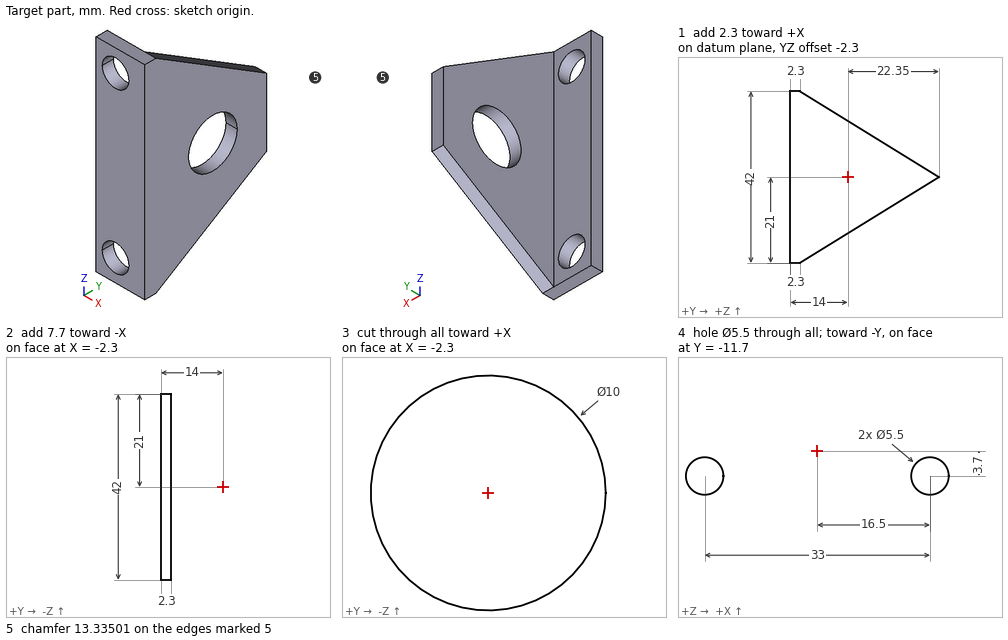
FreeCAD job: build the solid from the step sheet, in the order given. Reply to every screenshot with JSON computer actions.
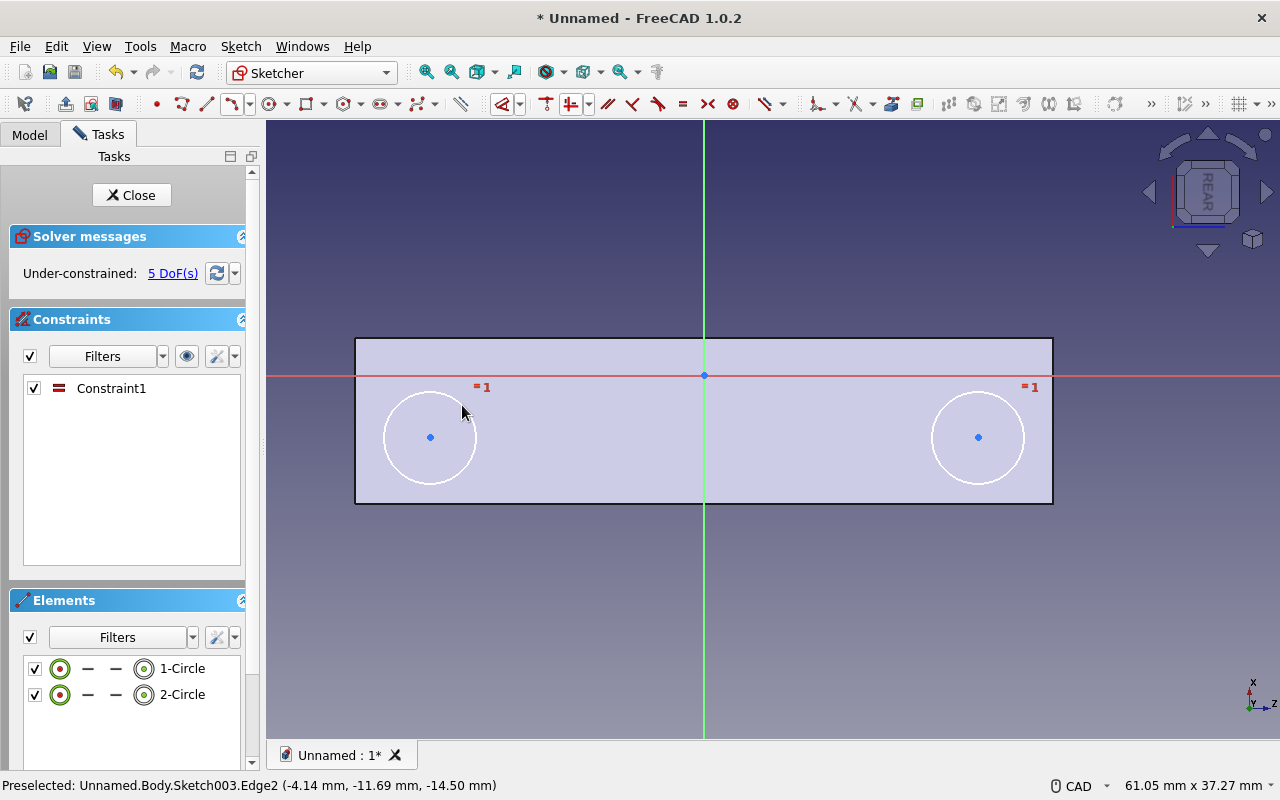
{"action": "left_click", "coordinate": [978, 438]}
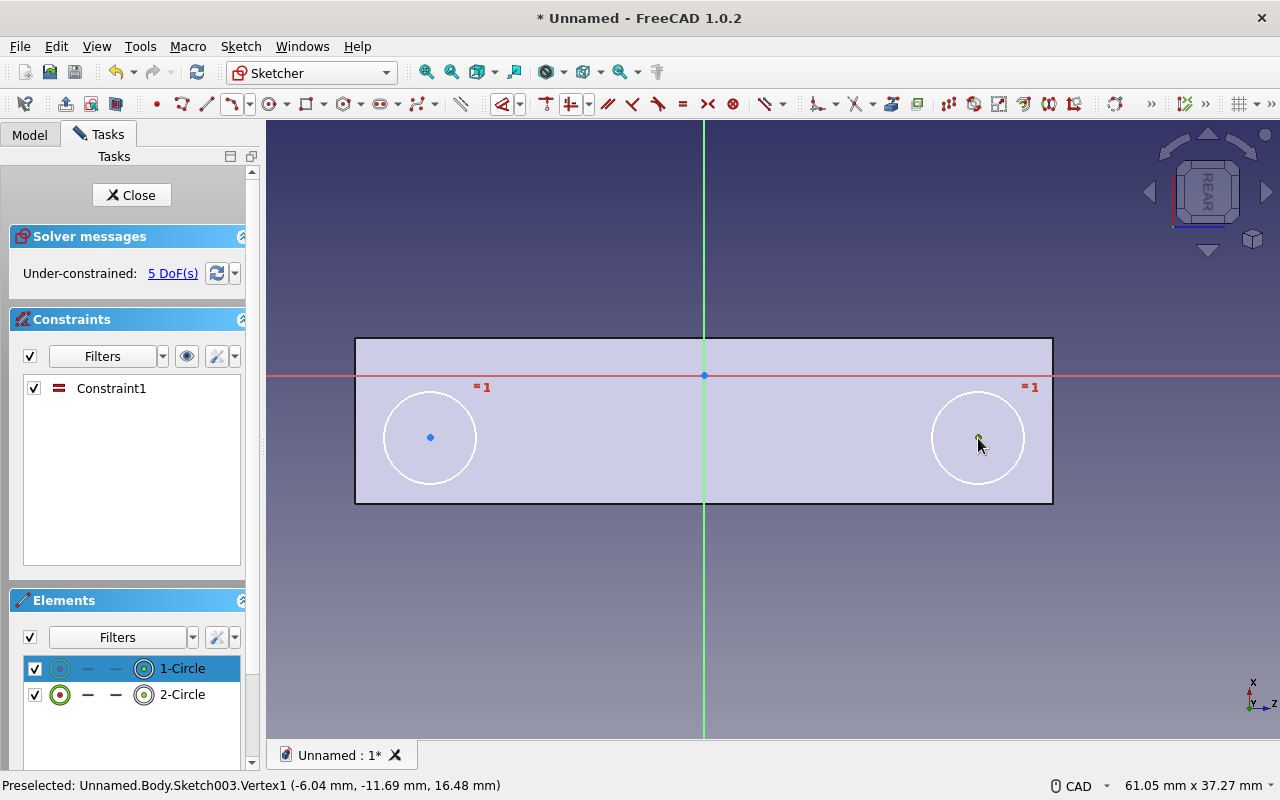
{"action": "left_click", "coordinate": [430, 438]}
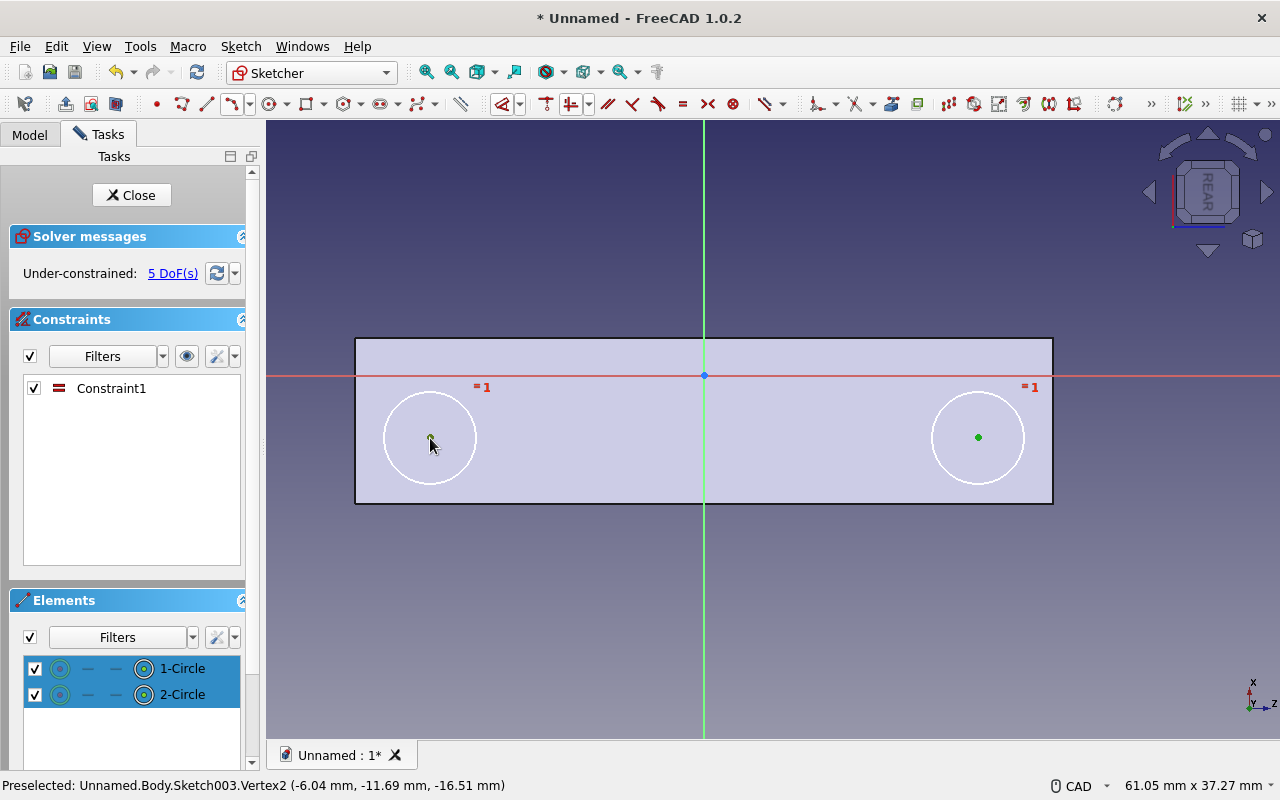
{"action": "key", "text": "h"}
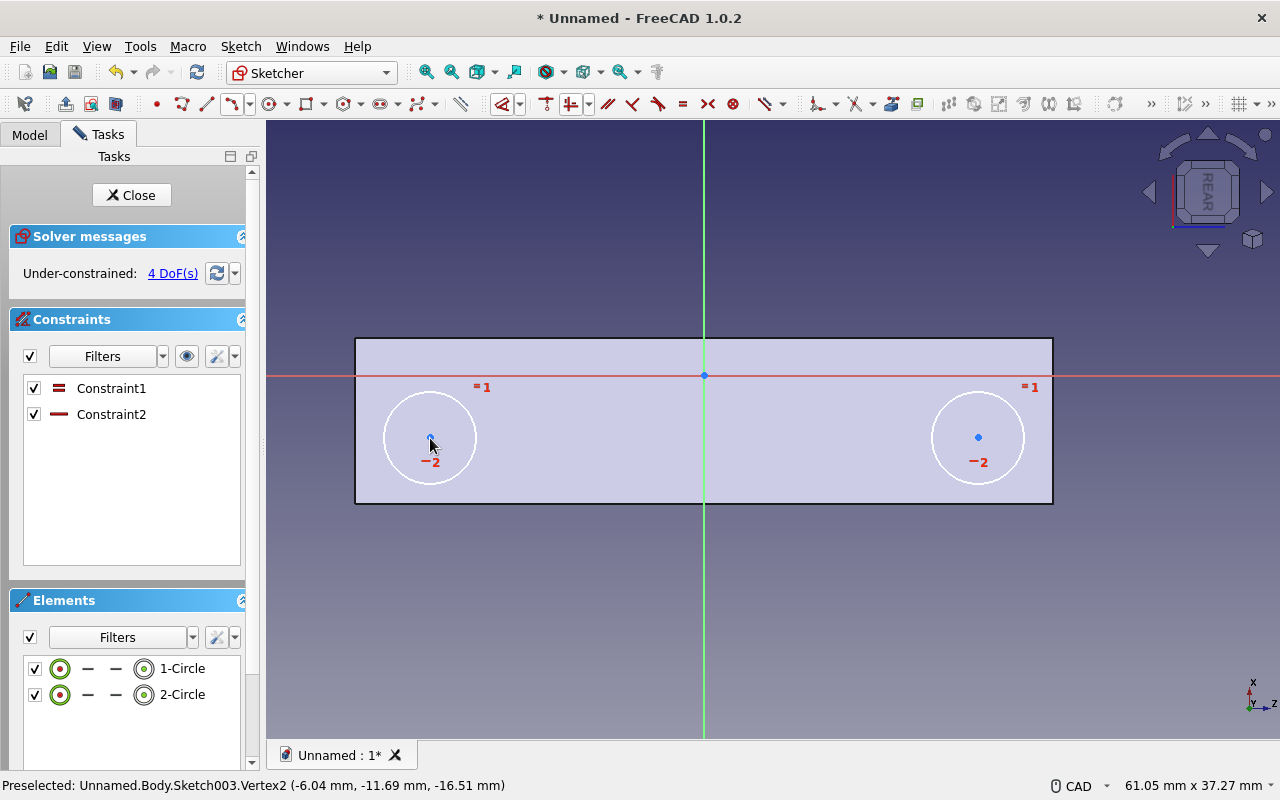
{"action": "left_click", "coordinate": [1010, 405]}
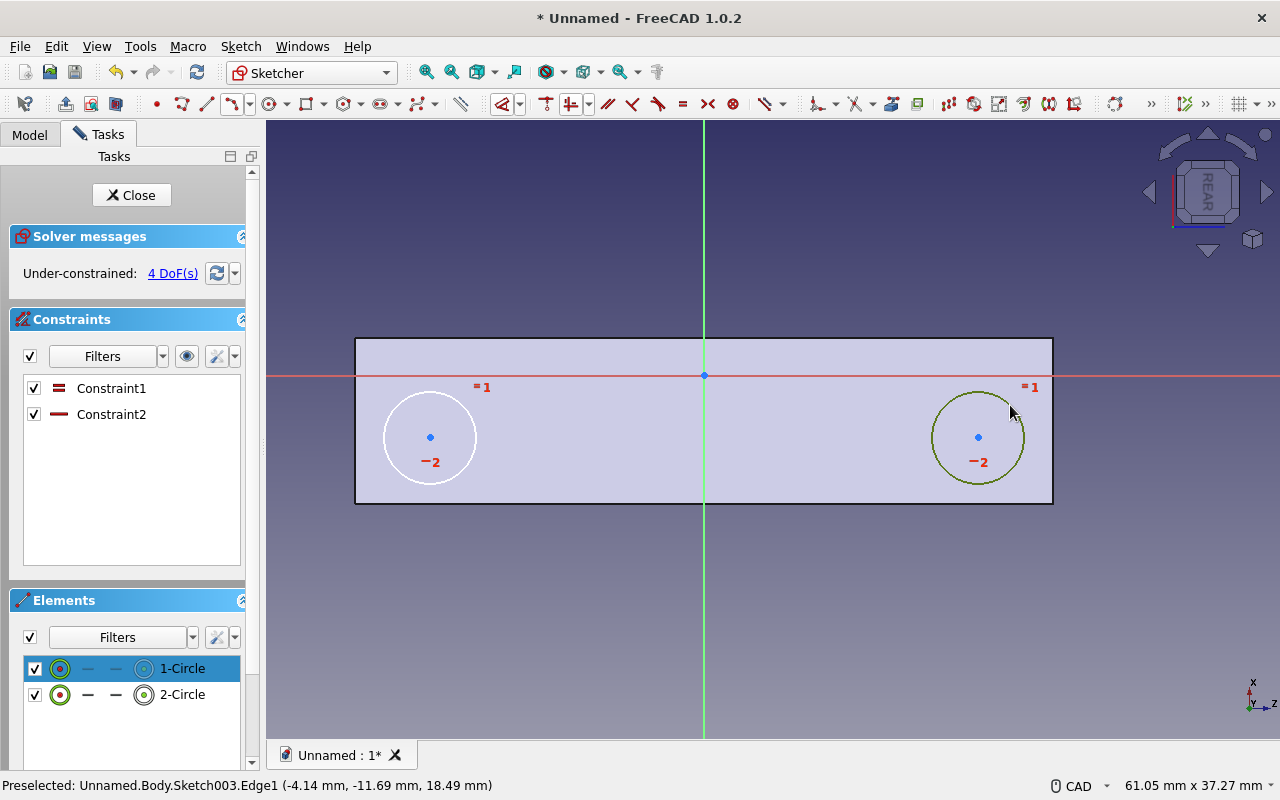
{"action": "left_click", "coordinate": [520, 104]}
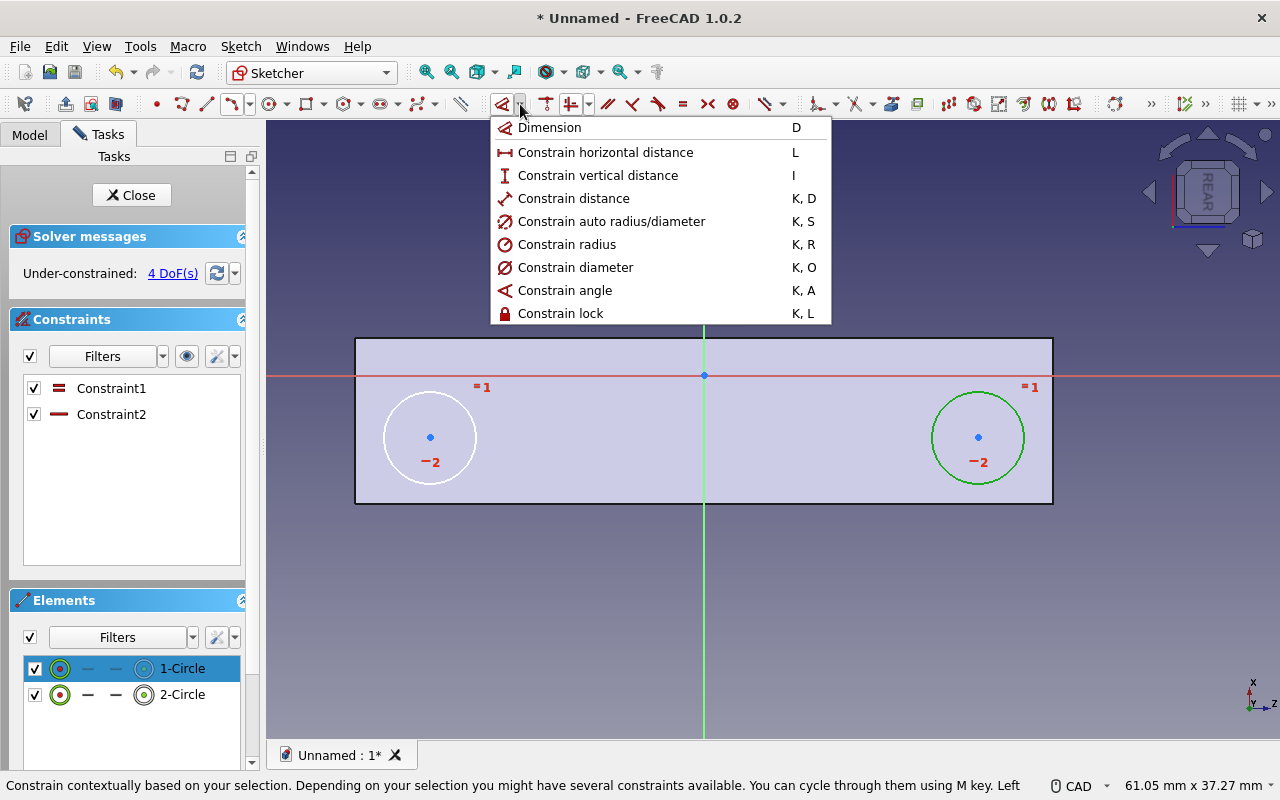
{"action": "left_click", "coordinate": [661, 268]}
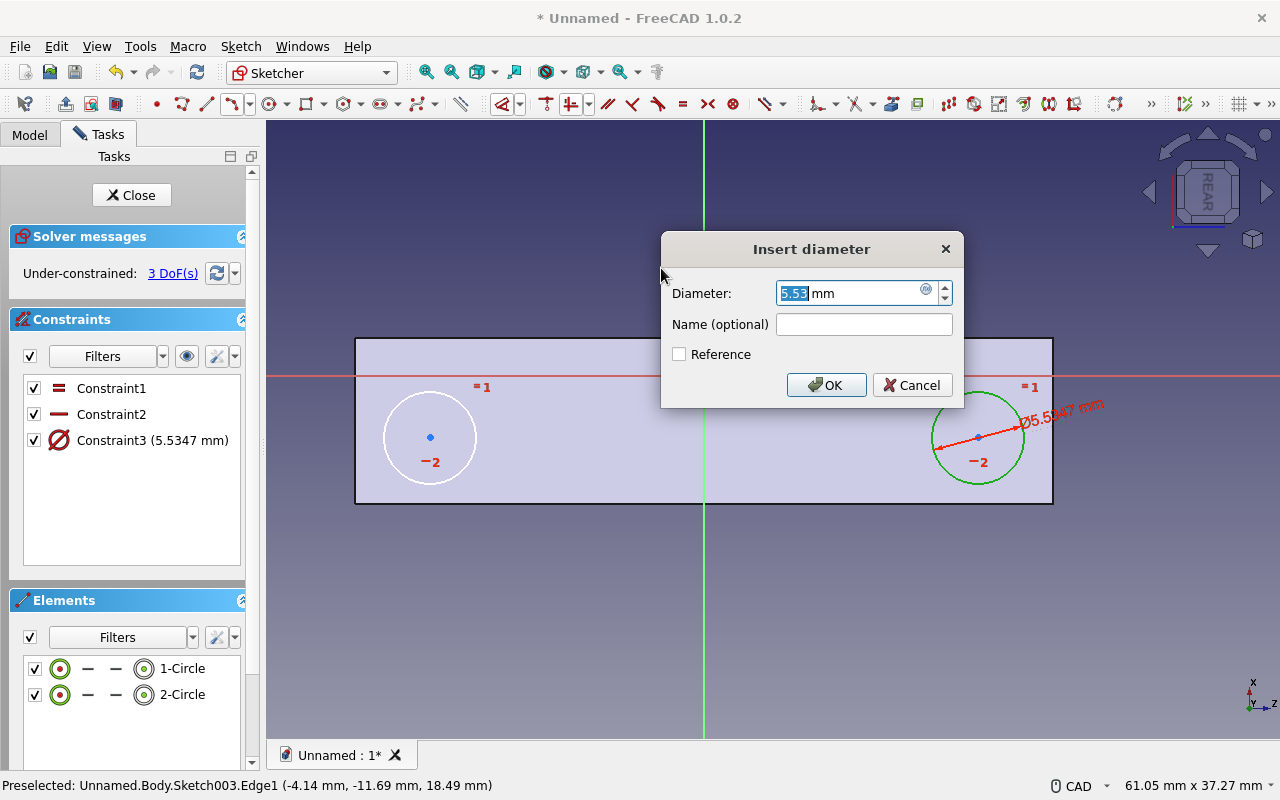
{"action": "type", "text": "5.5"}
{"action": "key", "text": "Return"}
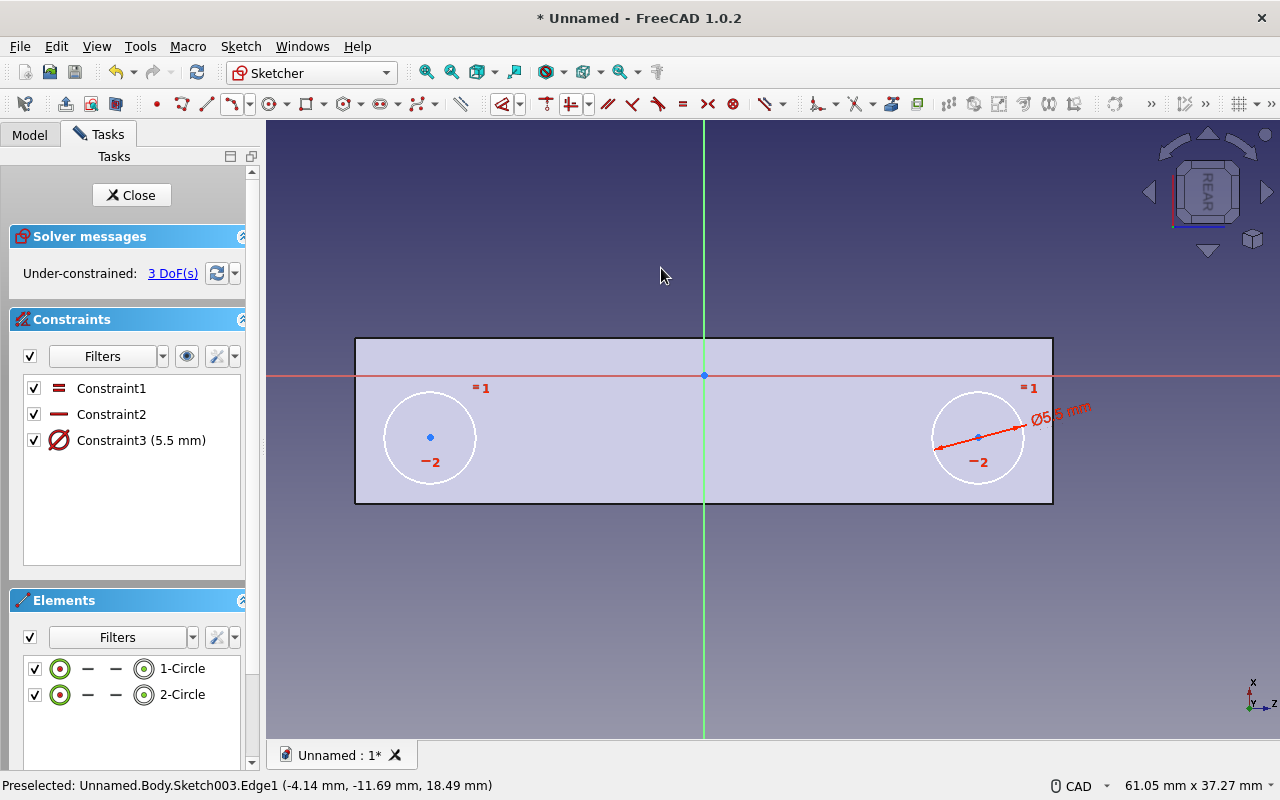
{"action": "left_click", "coordinate": [978, 438]}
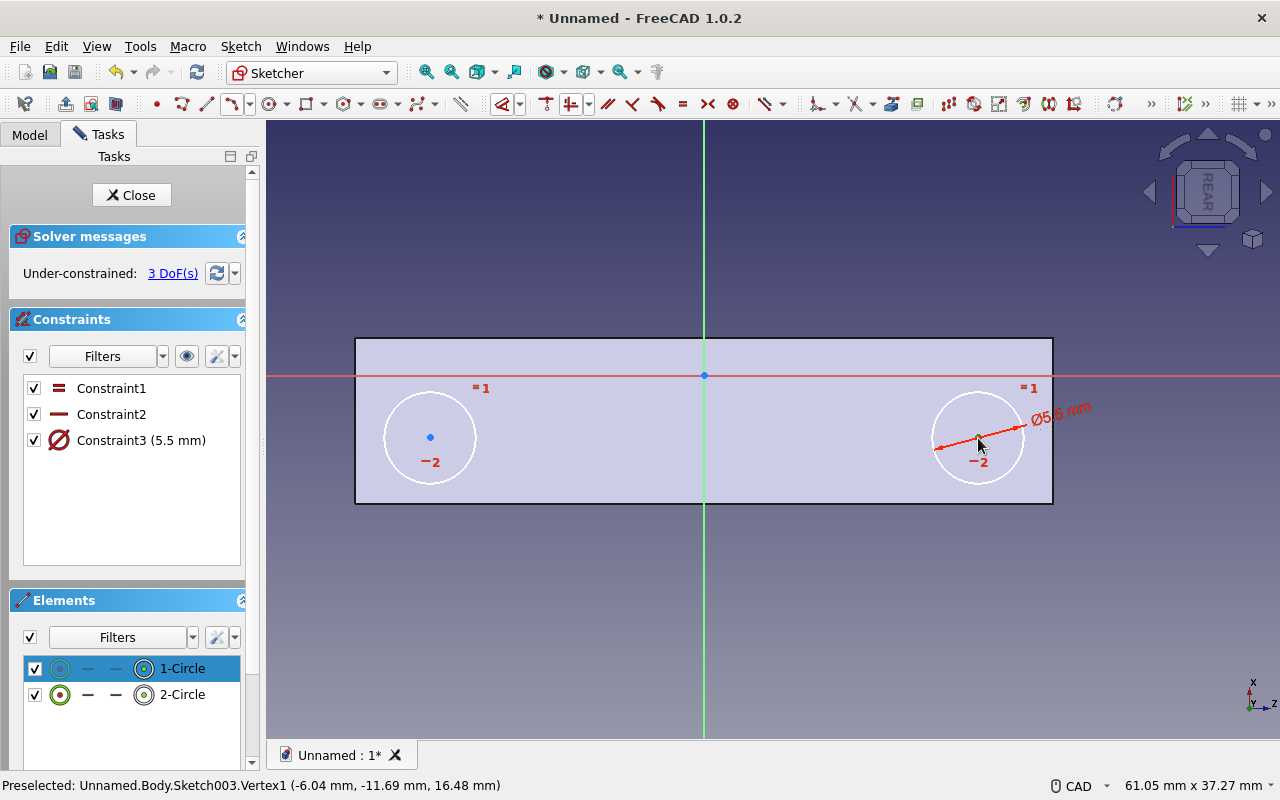
{"action": "key", "text": "i"}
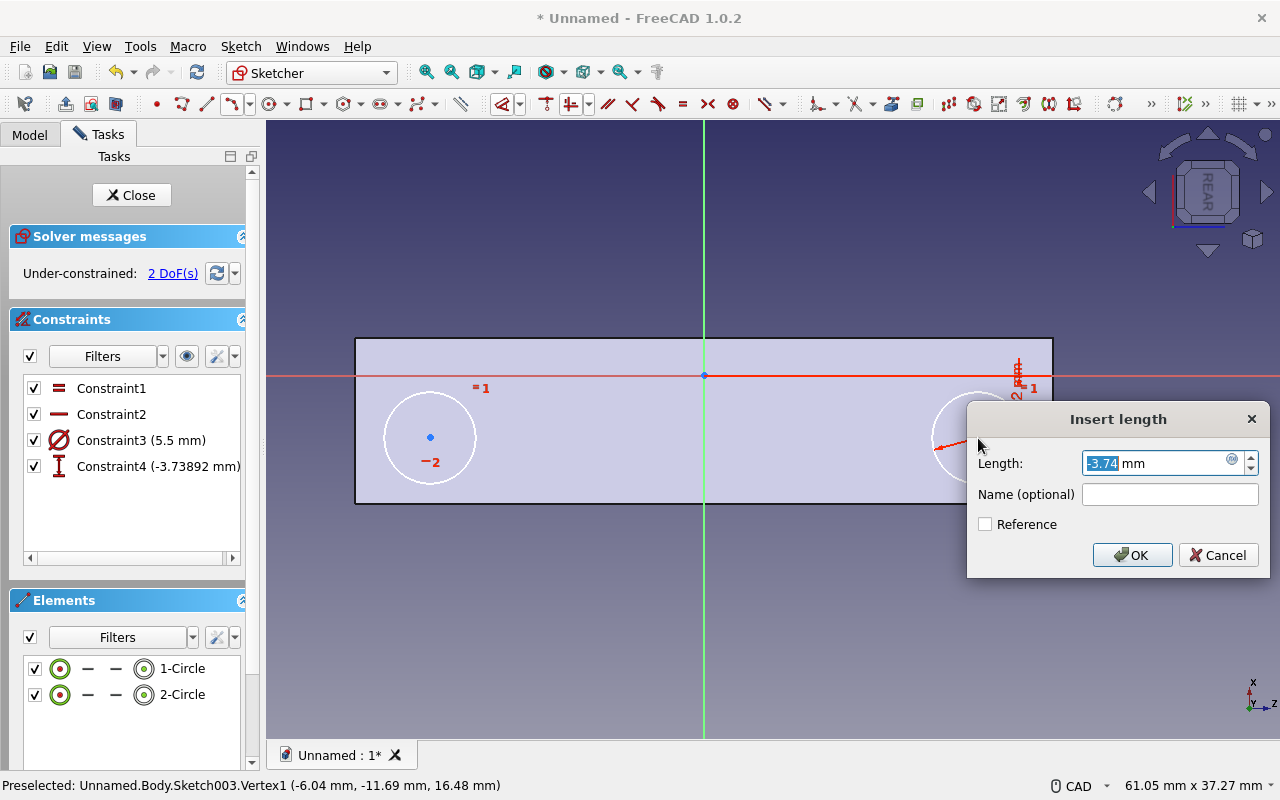
{"action": "type", "text": "-3.7"}
{"action": "key", "text": "Return"}